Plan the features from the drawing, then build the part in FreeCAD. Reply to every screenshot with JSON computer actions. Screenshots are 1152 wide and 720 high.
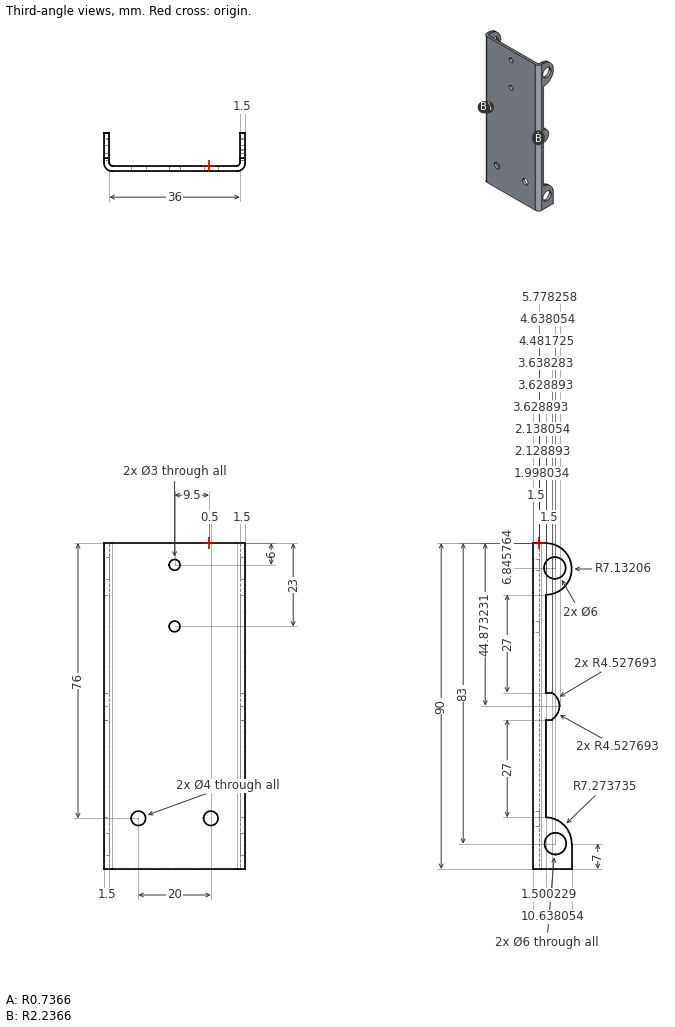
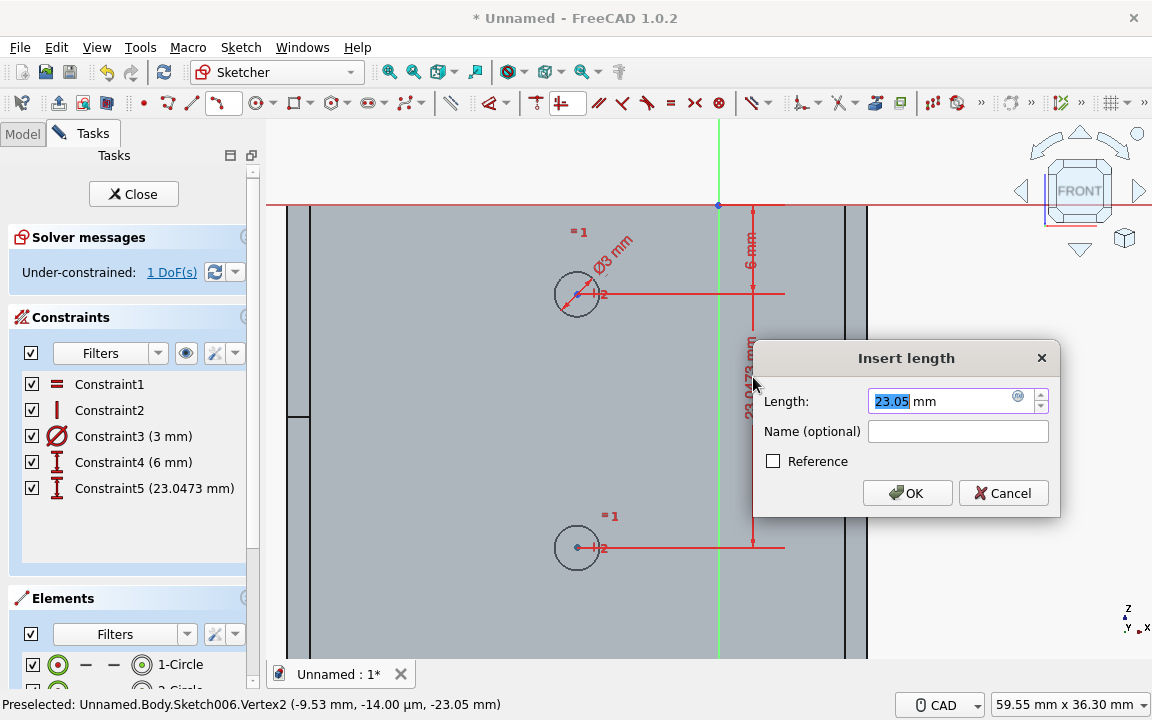
{"action": "type", "text": "23"}
{"action": "key", "text": "Return"}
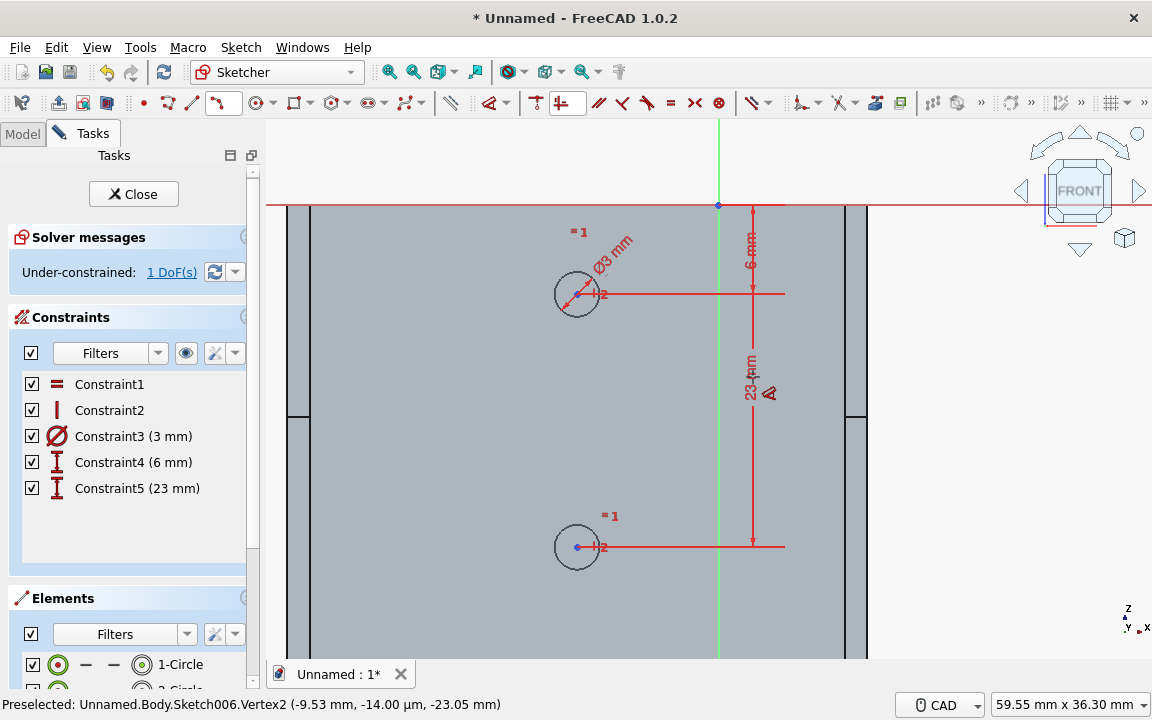
{"action": "left_click", "coordinate": [577, 294]}
{"action": "left_click", "coordinate": [648, 171]}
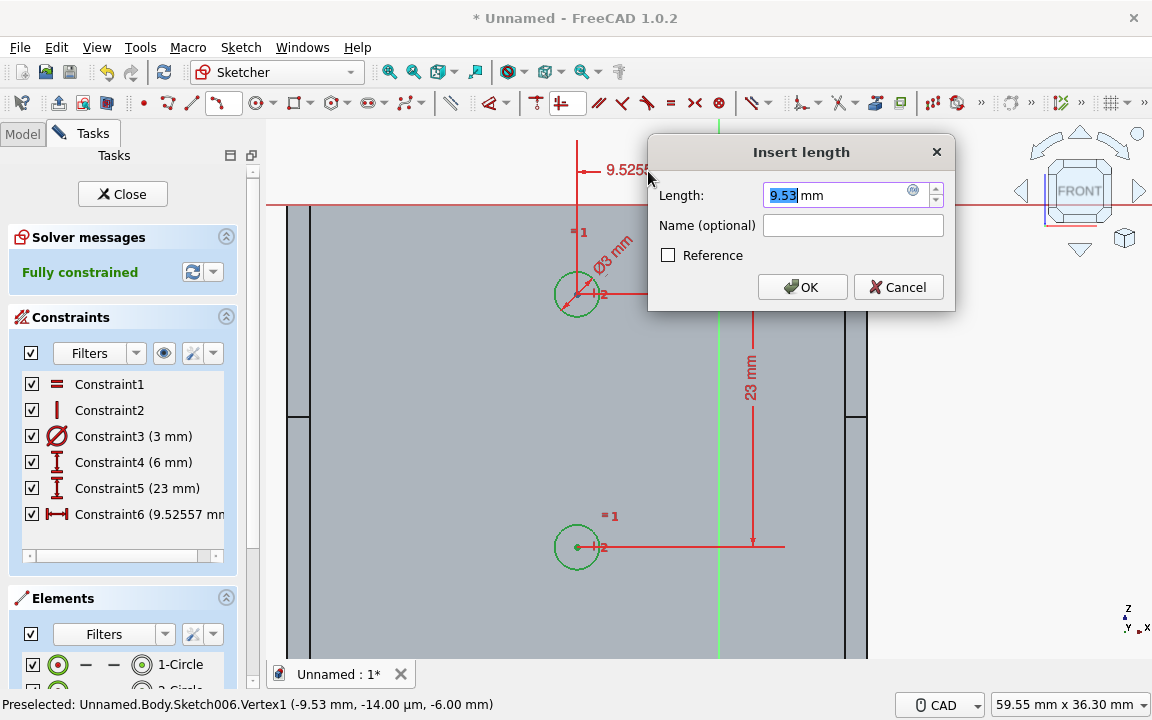
{"action": "type", "text": "9.5"}
{"action": "key", "text": "Return"}
{"action": "key", "text": "Escape"}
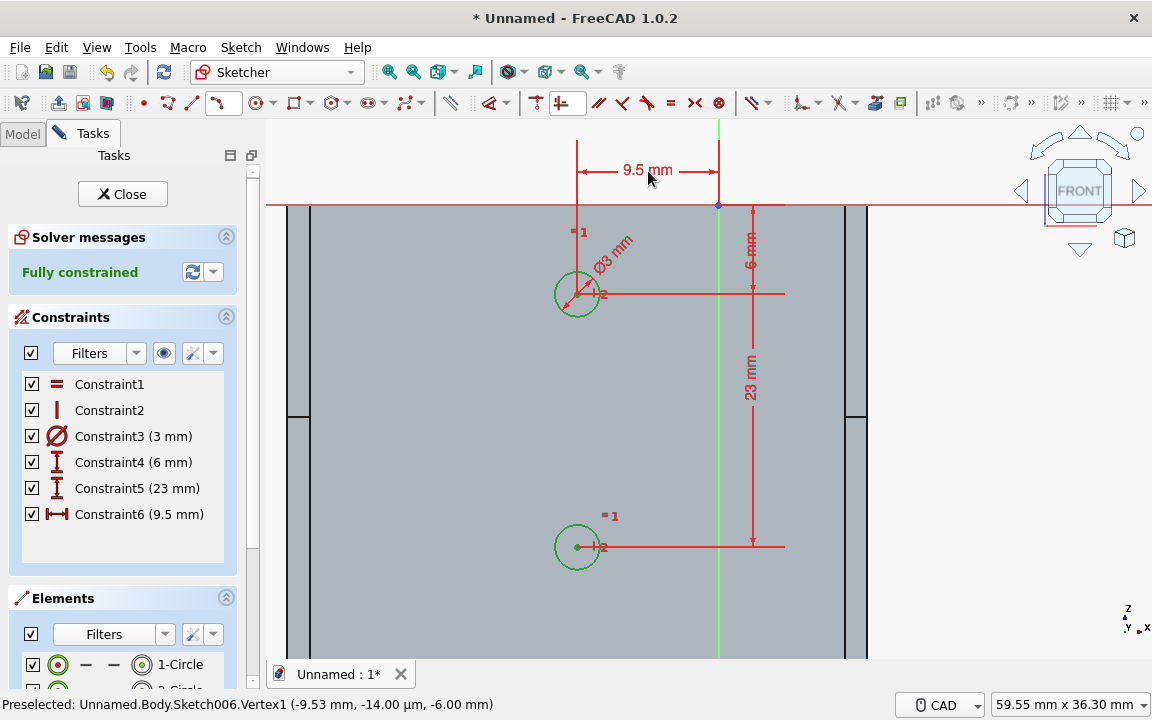
{"action": "left_click", "coordinate": [123, 194]}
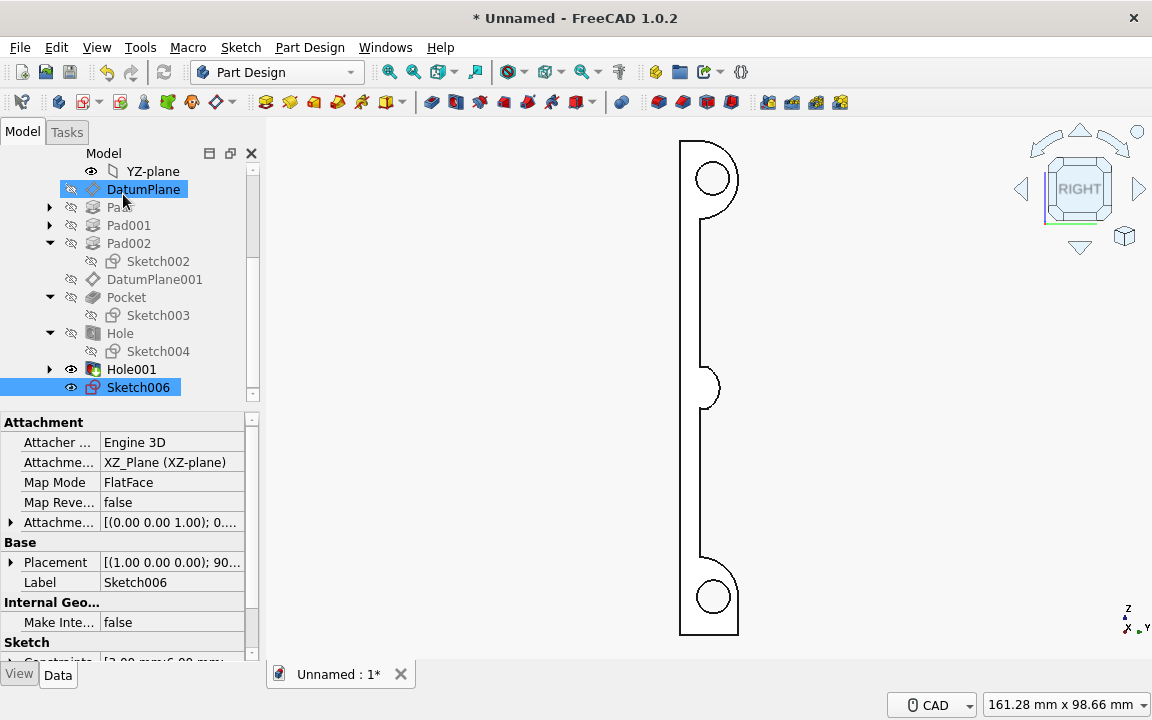
{"action": "left_click", "coordinate": [456, 102]}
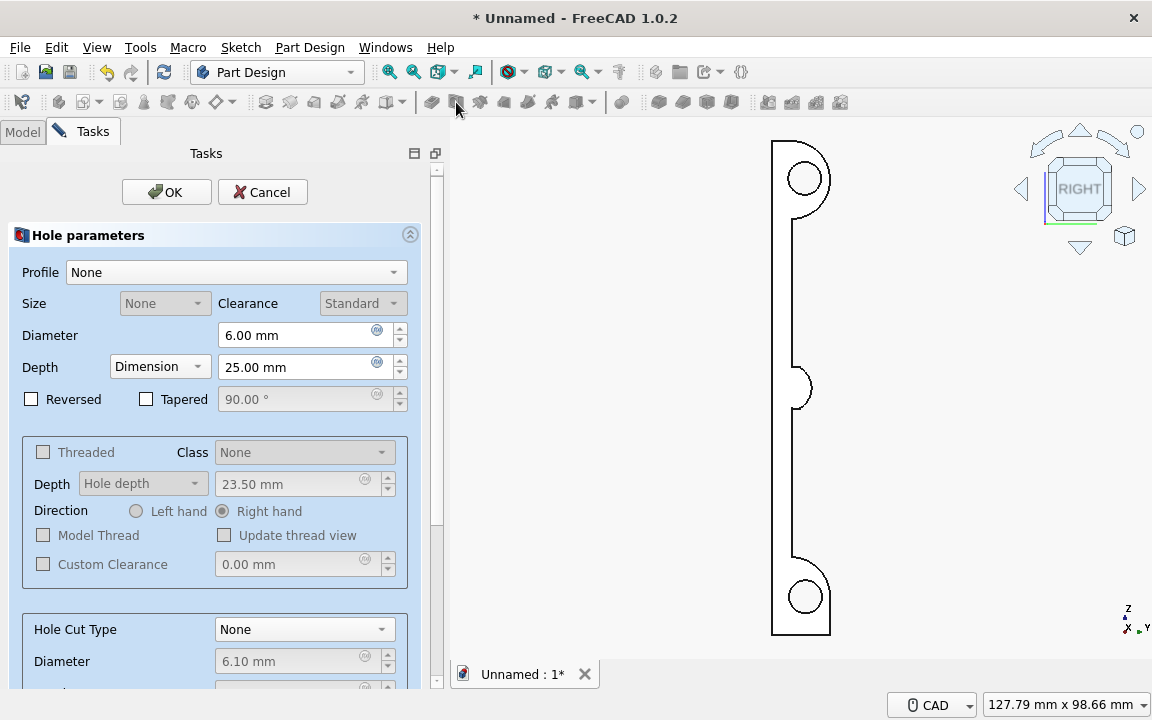
{"action": "triple_click", "coordinate": [305, 335]}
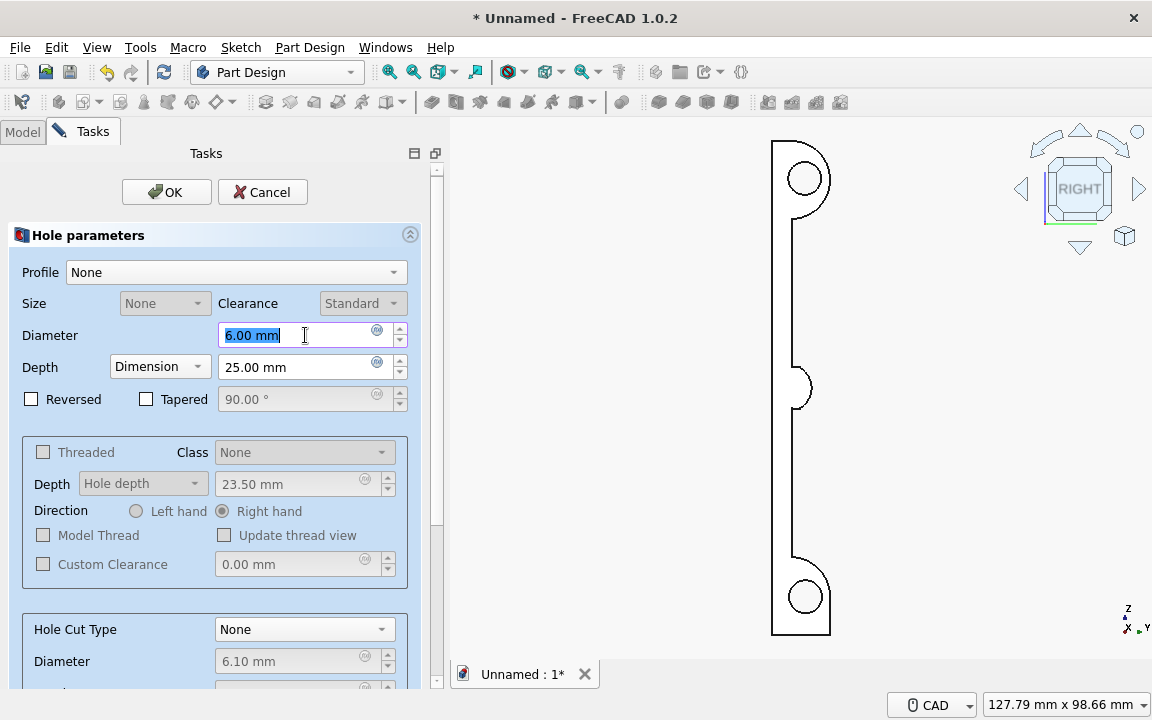
{"action": "type", "text": "3"}
{"action": "key", "text": "Tab"}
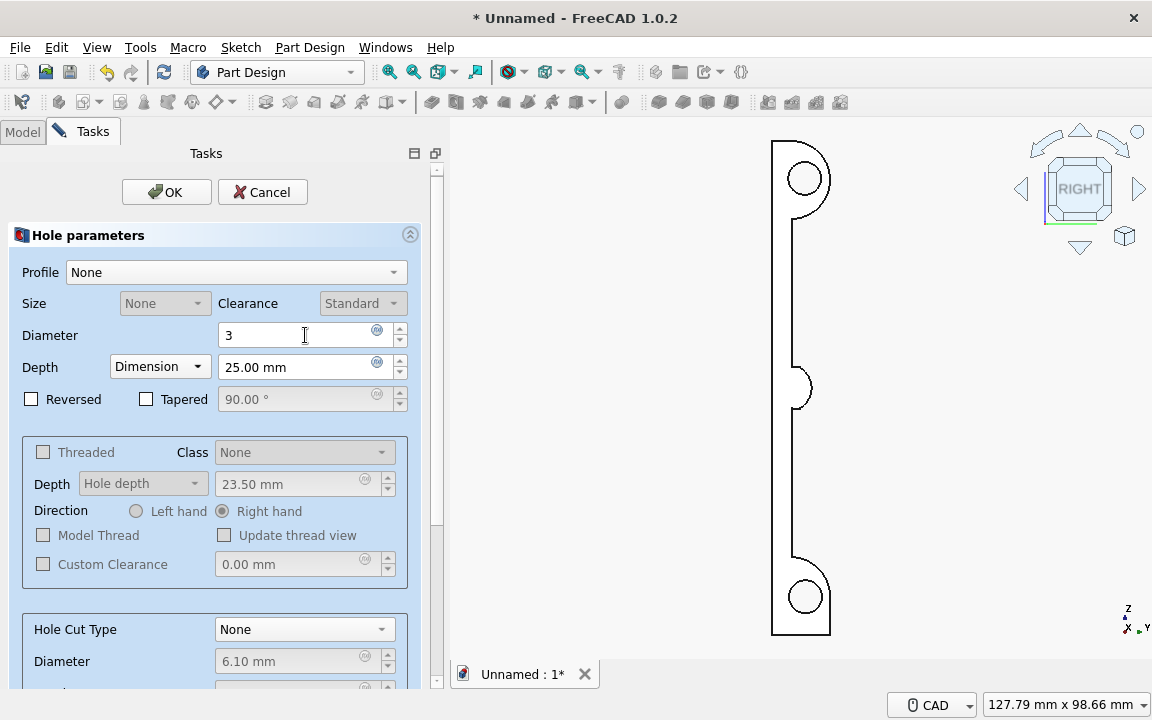
{"action": "left_click", "coordinate": [161, 366]}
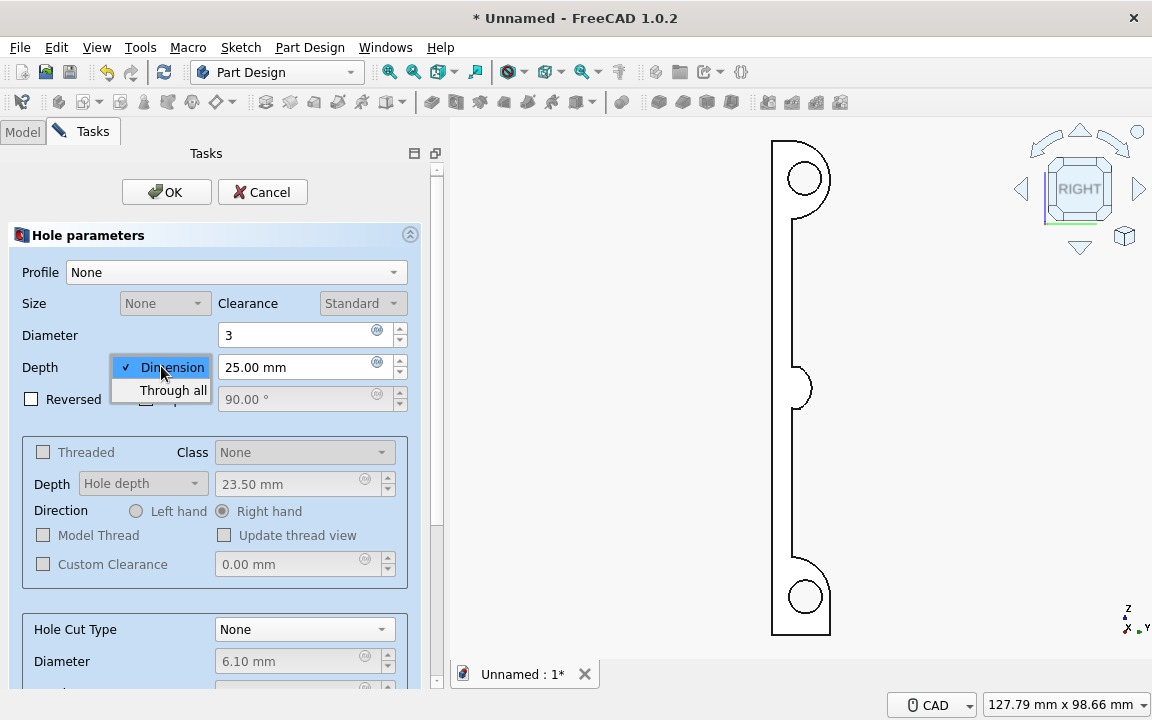
{"action": "left_click", "coordinate": [160, 390]}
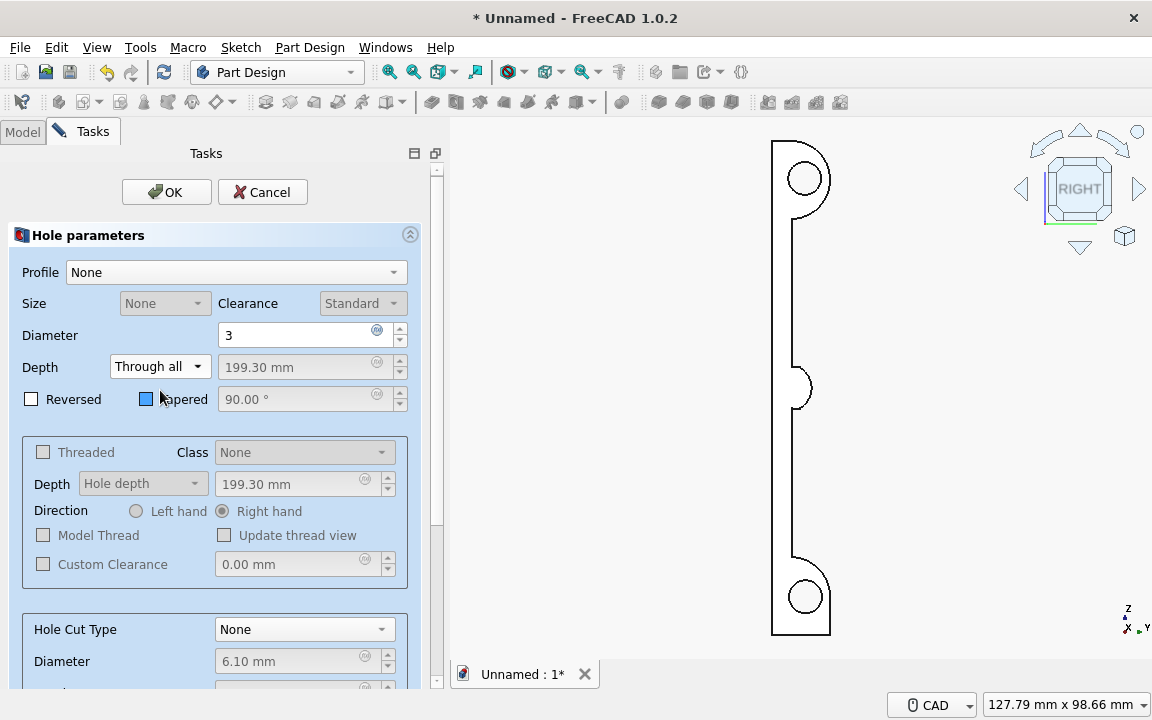
{"action": "left_click", "coordinate": [30, 399]}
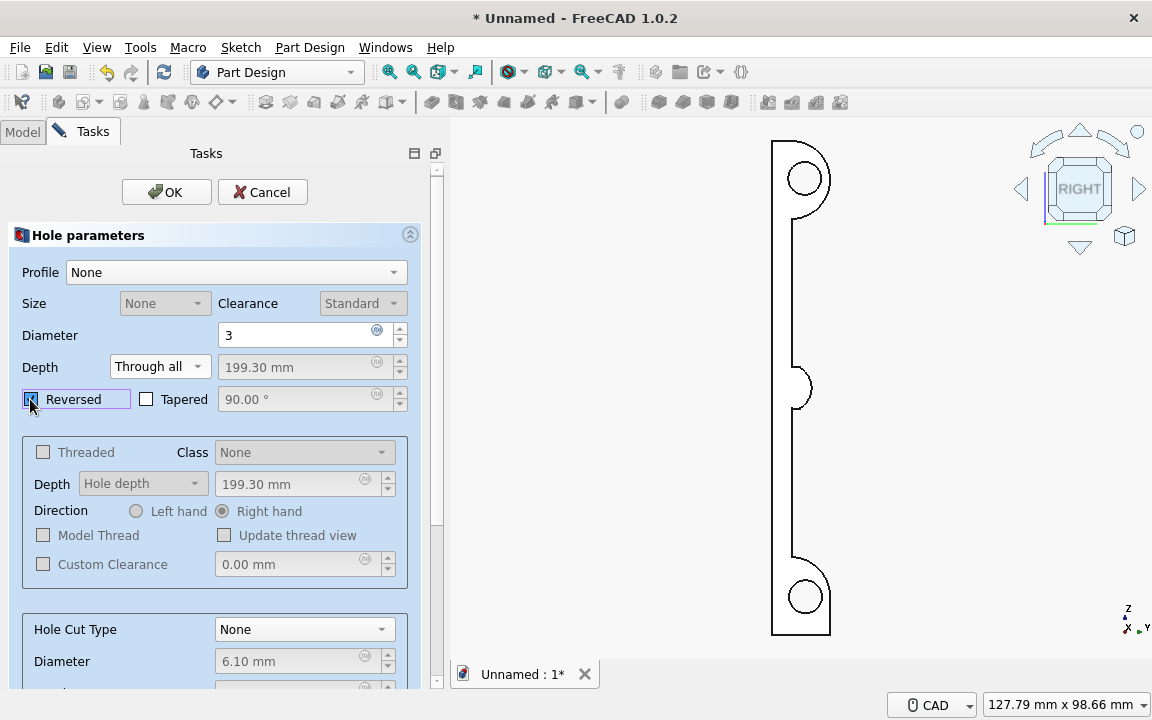
{"action": "left_click", "coordinate": [167, 192]}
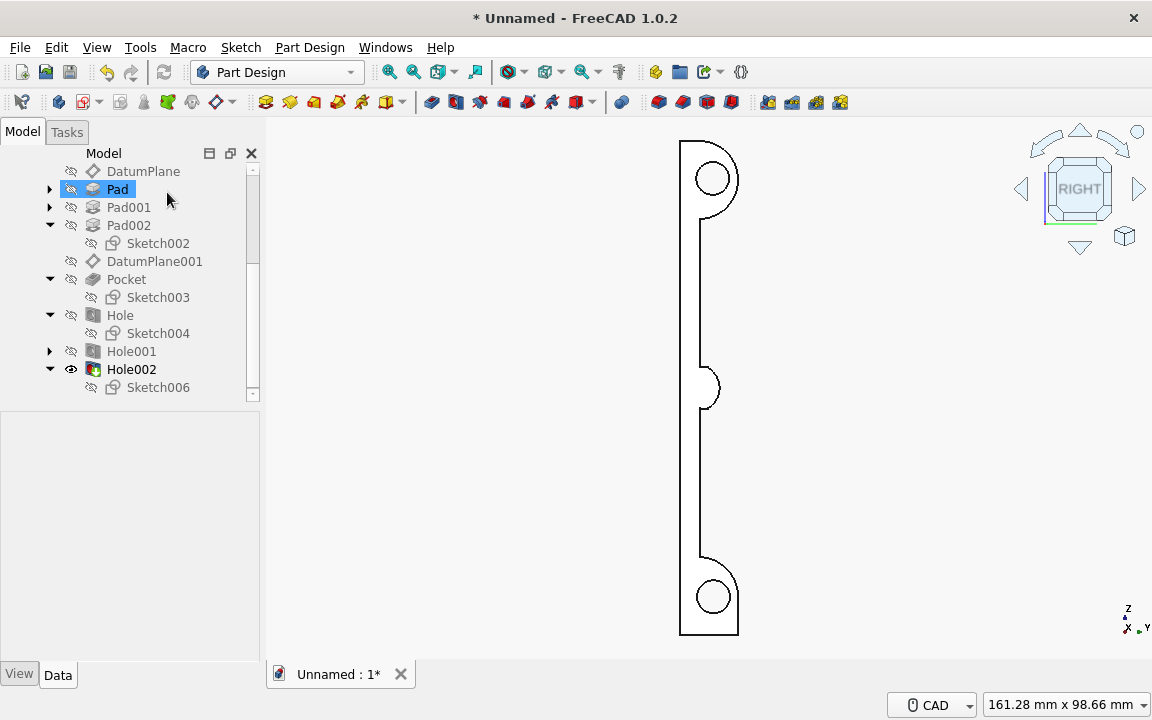
{"action": "key", "text": "0"}